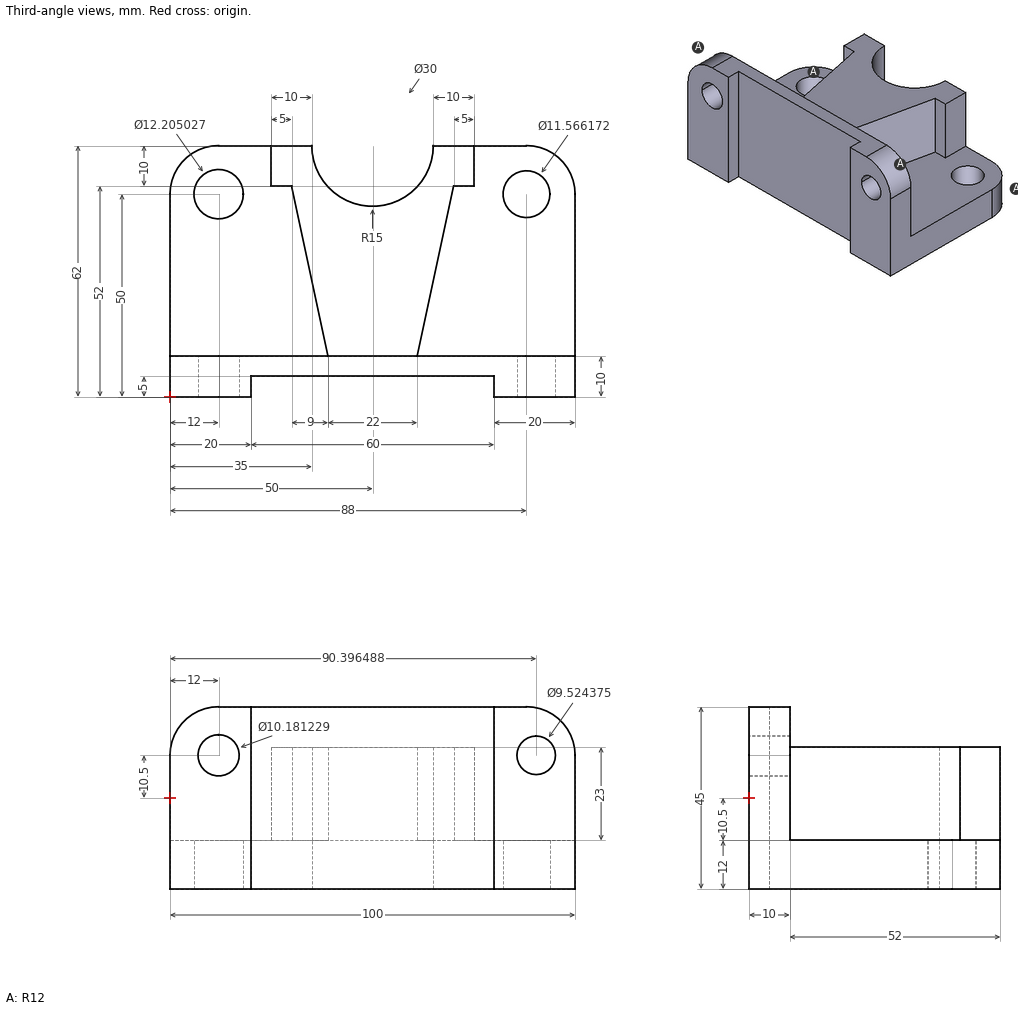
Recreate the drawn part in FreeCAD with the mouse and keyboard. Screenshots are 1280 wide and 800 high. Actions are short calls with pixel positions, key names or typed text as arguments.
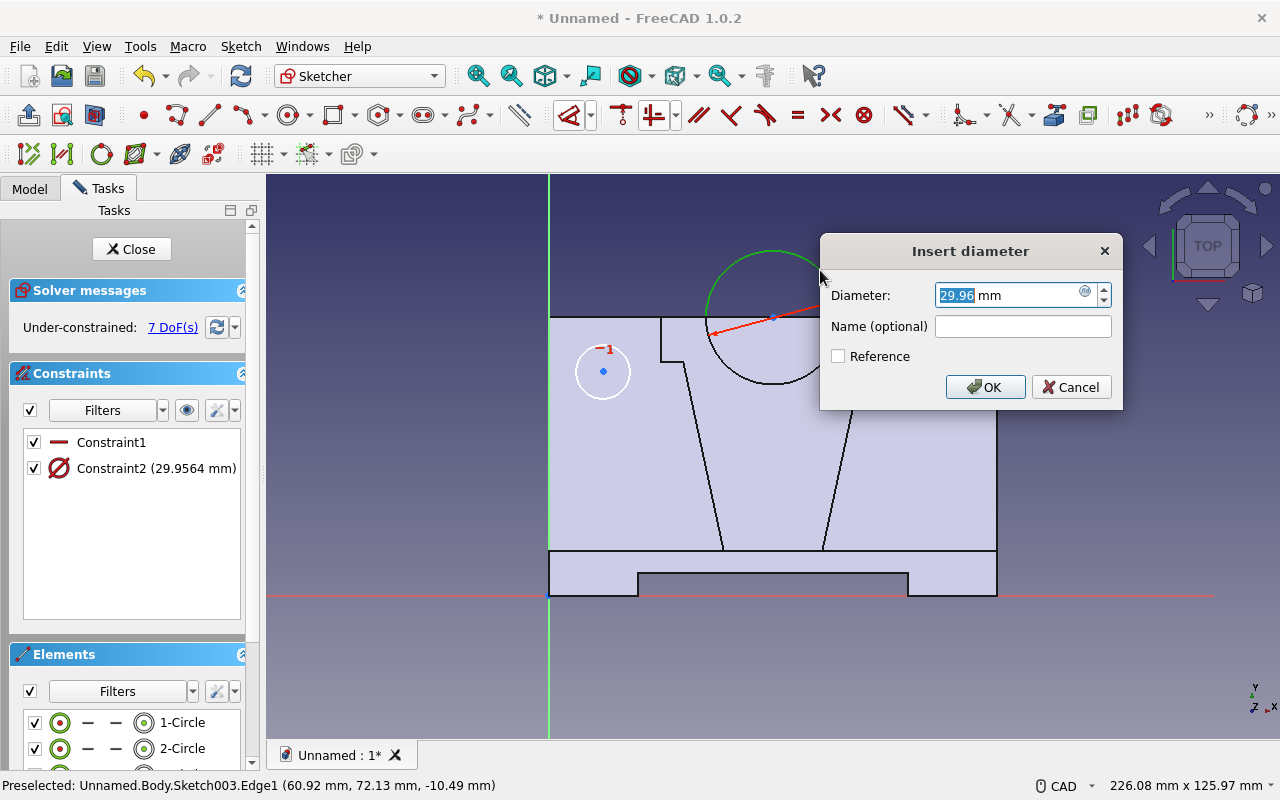
text(30)
key(Return)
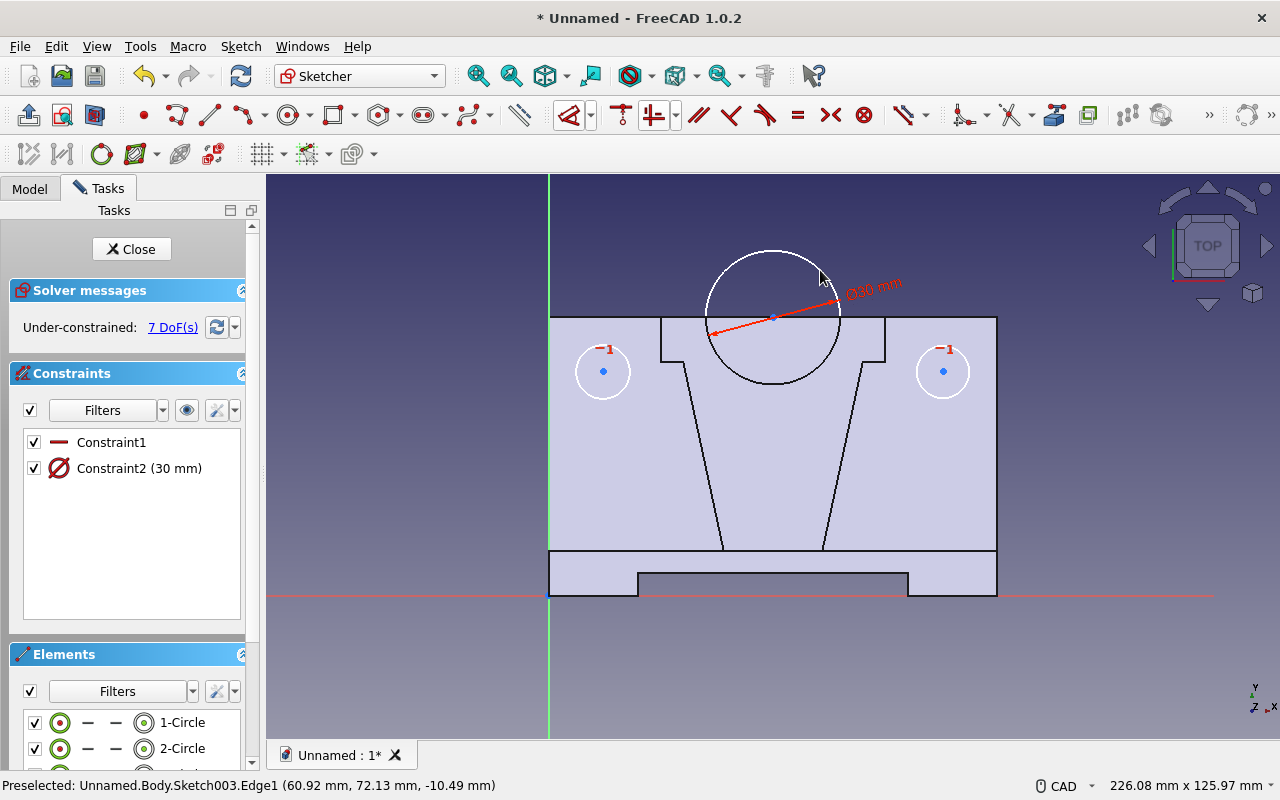
click(622, 353)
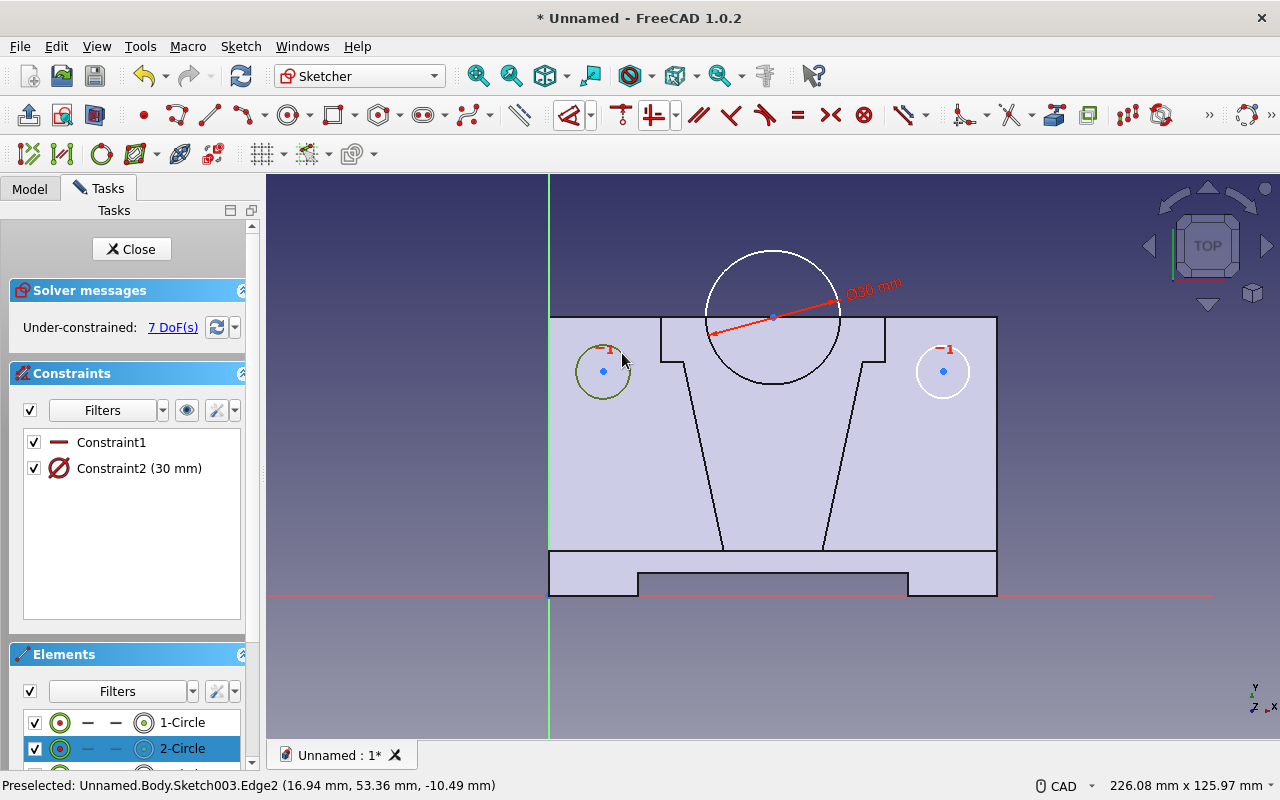
click(590, 116)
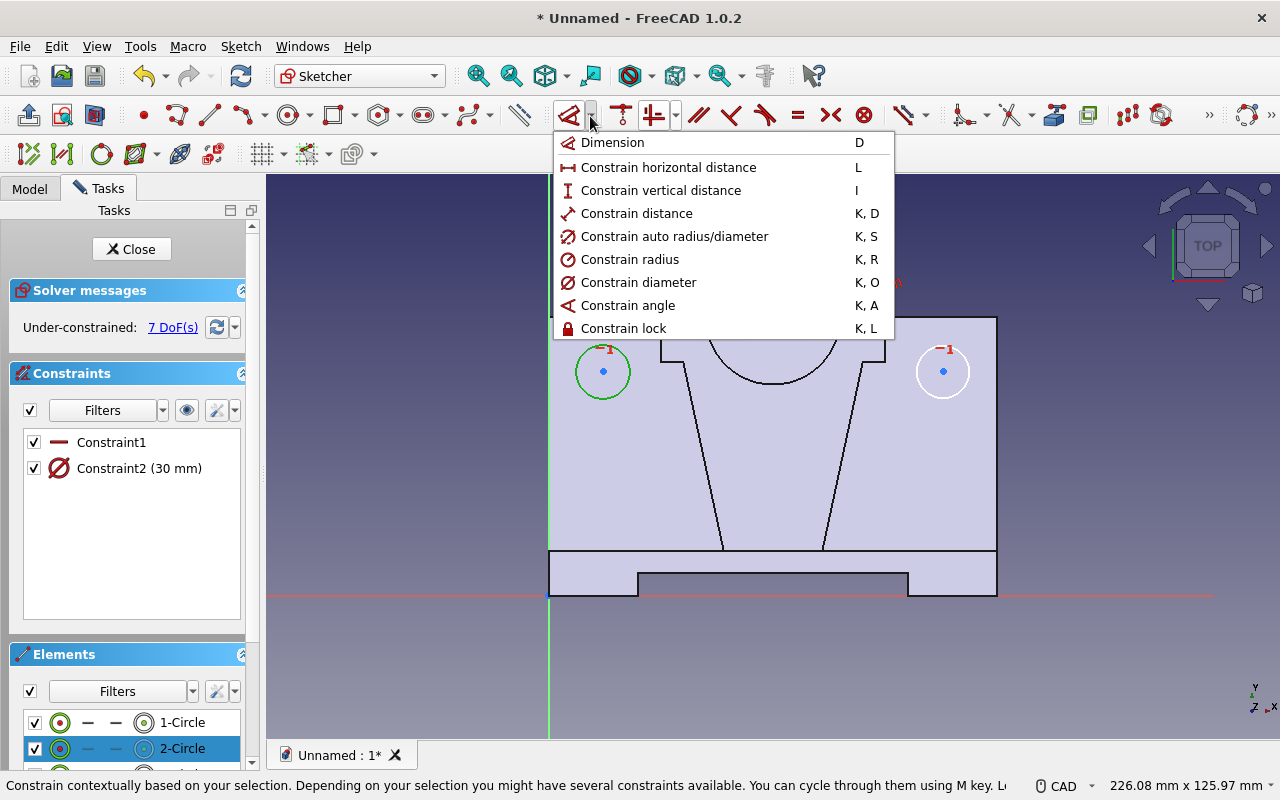
click(724, 282)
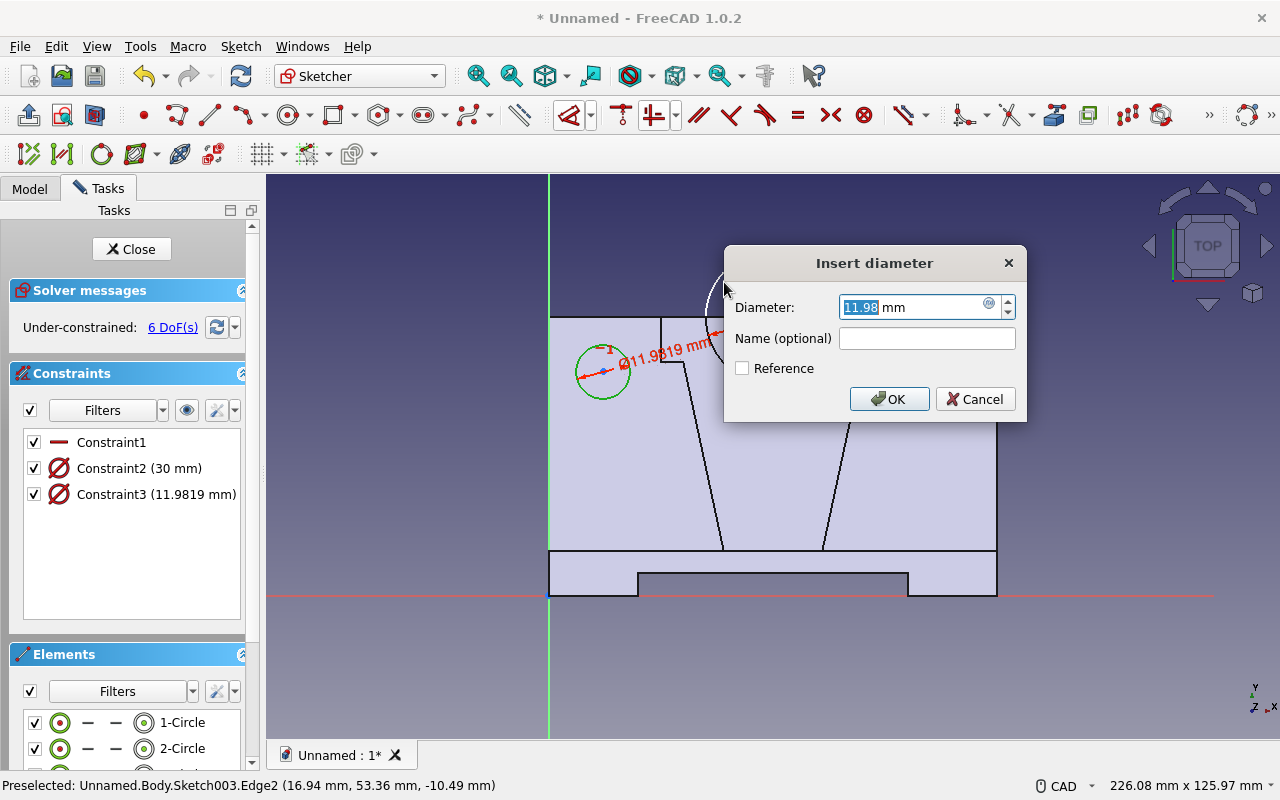
text(12.205027)
key(Return)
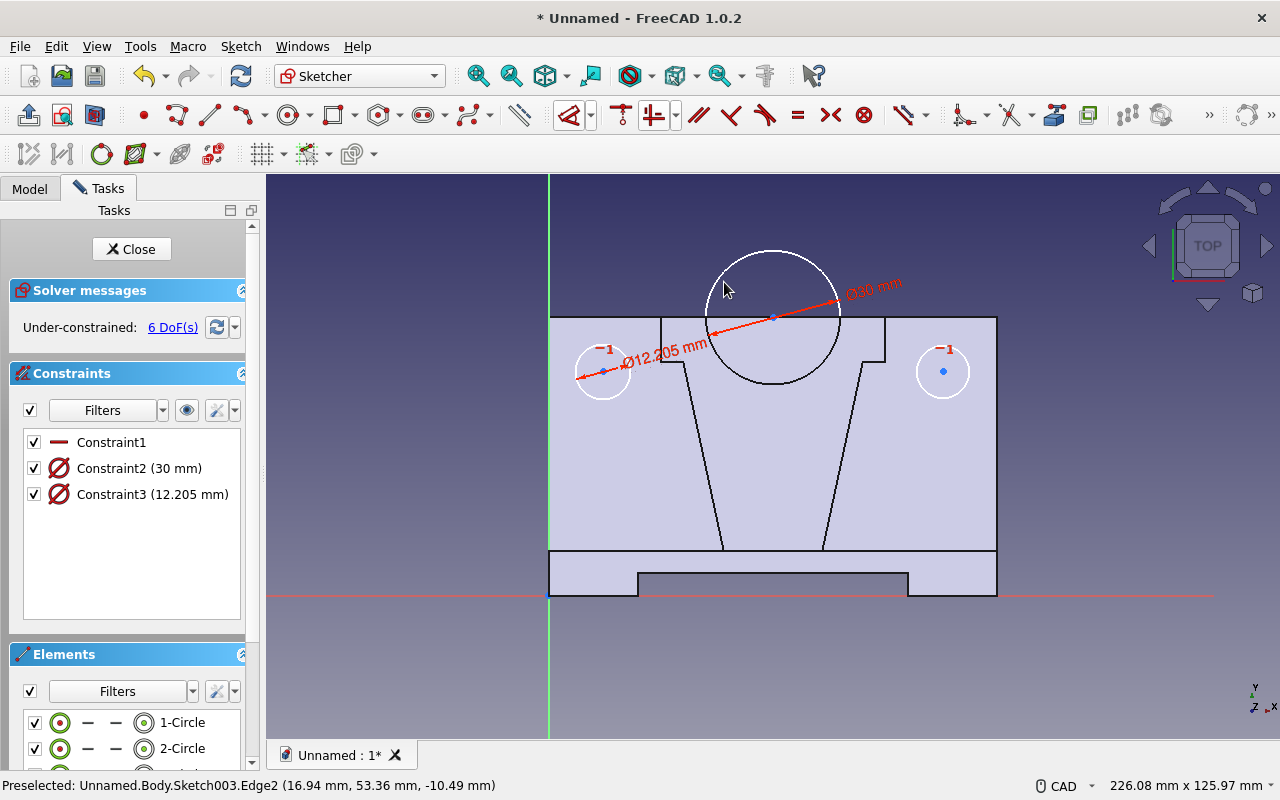
click(961, 353)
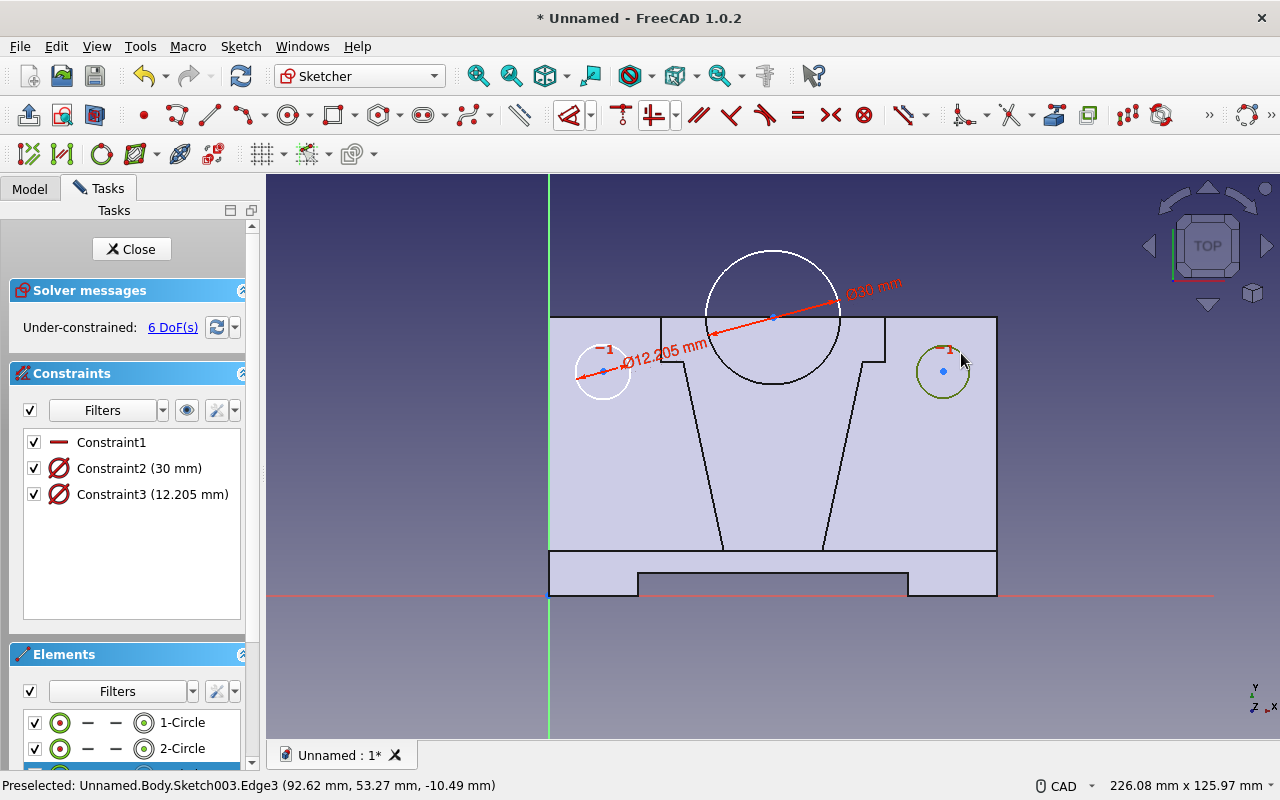
key(k)
key(o)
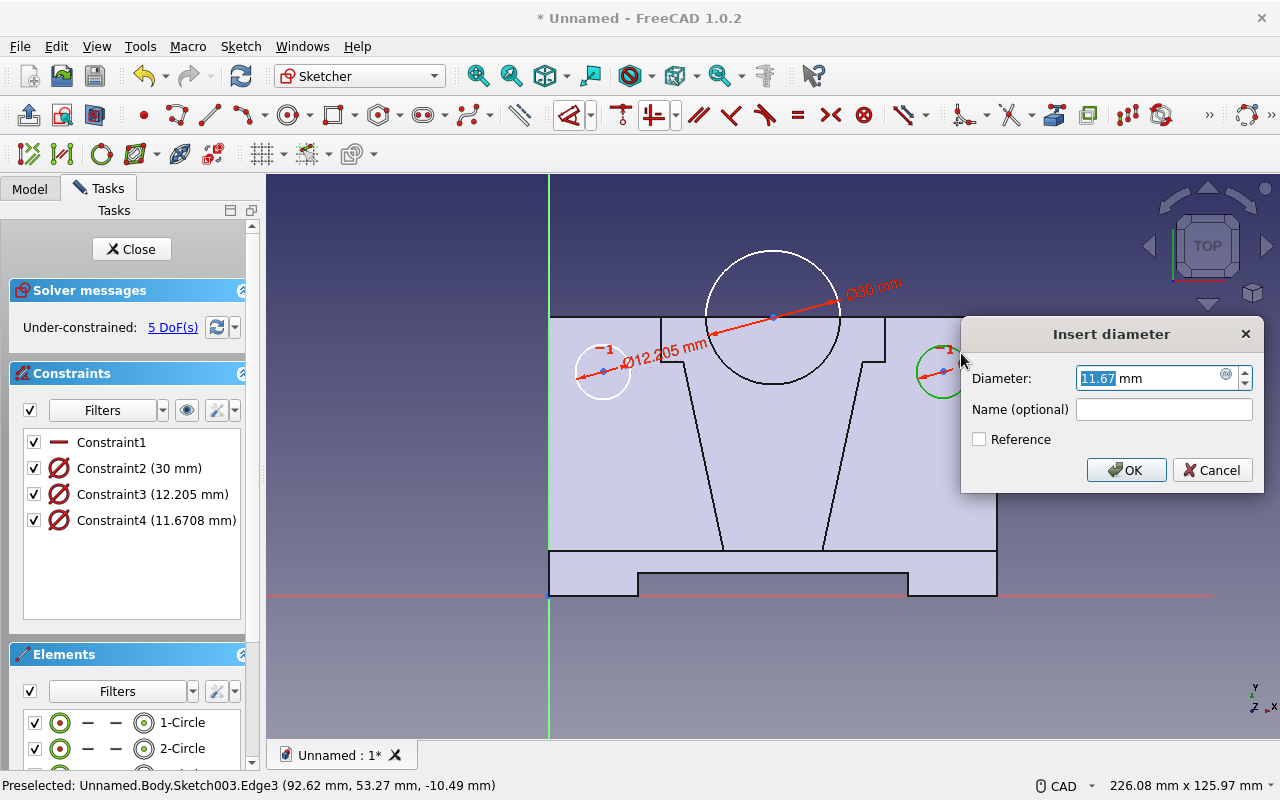
text(11.566172)
key(Return)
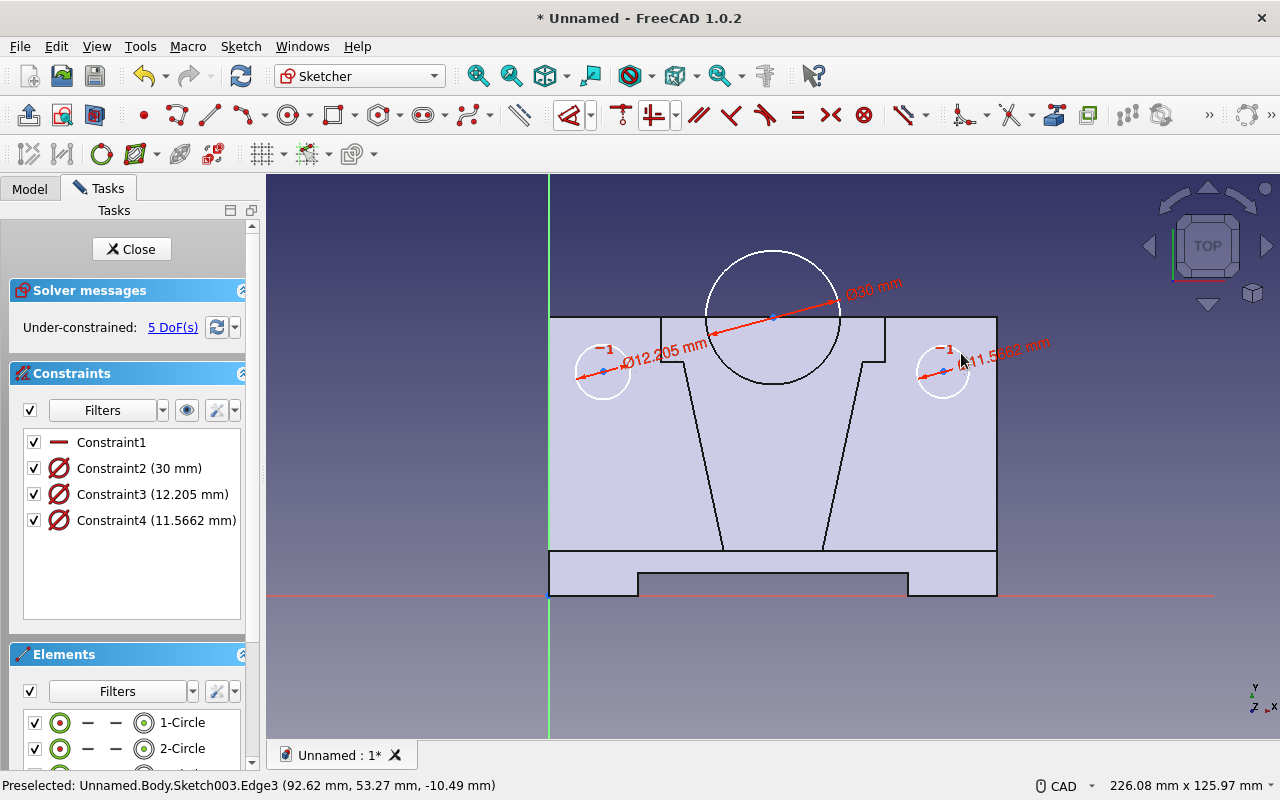
click(773, 318)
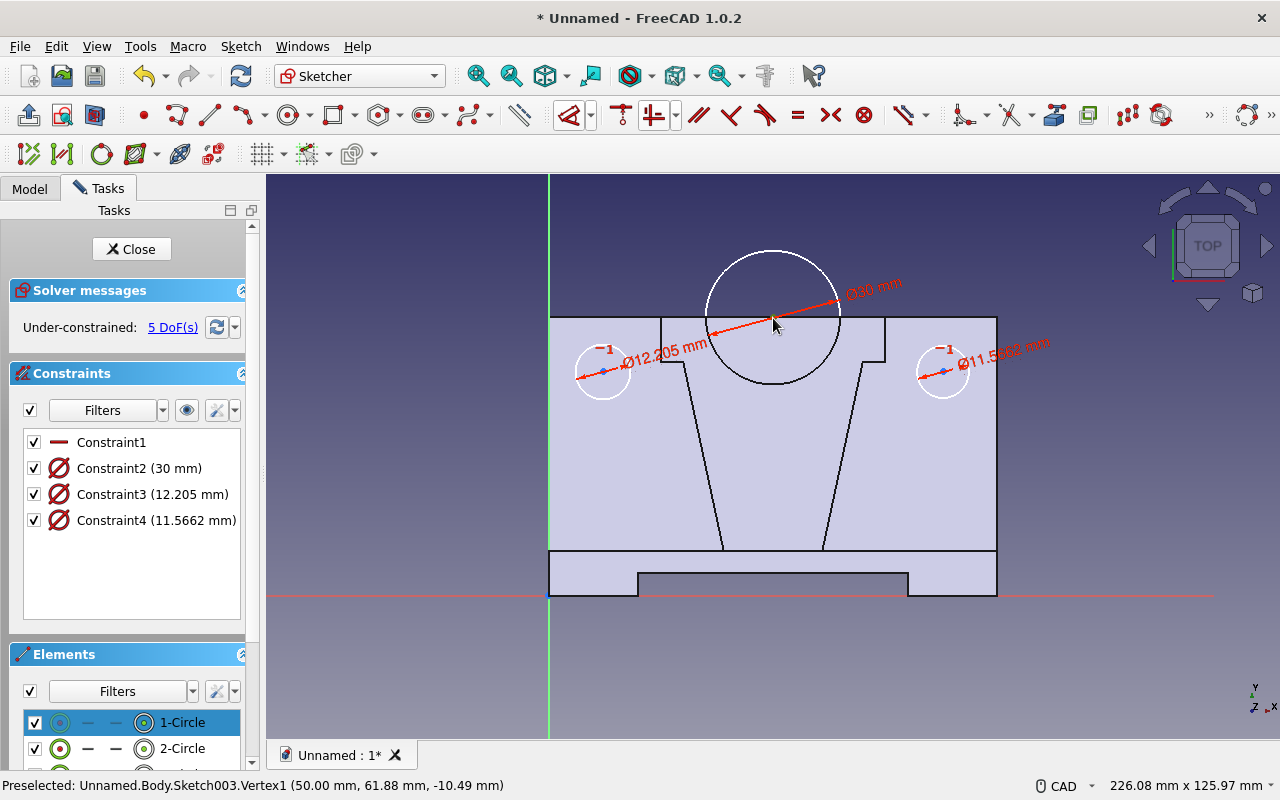
click(590, 116)